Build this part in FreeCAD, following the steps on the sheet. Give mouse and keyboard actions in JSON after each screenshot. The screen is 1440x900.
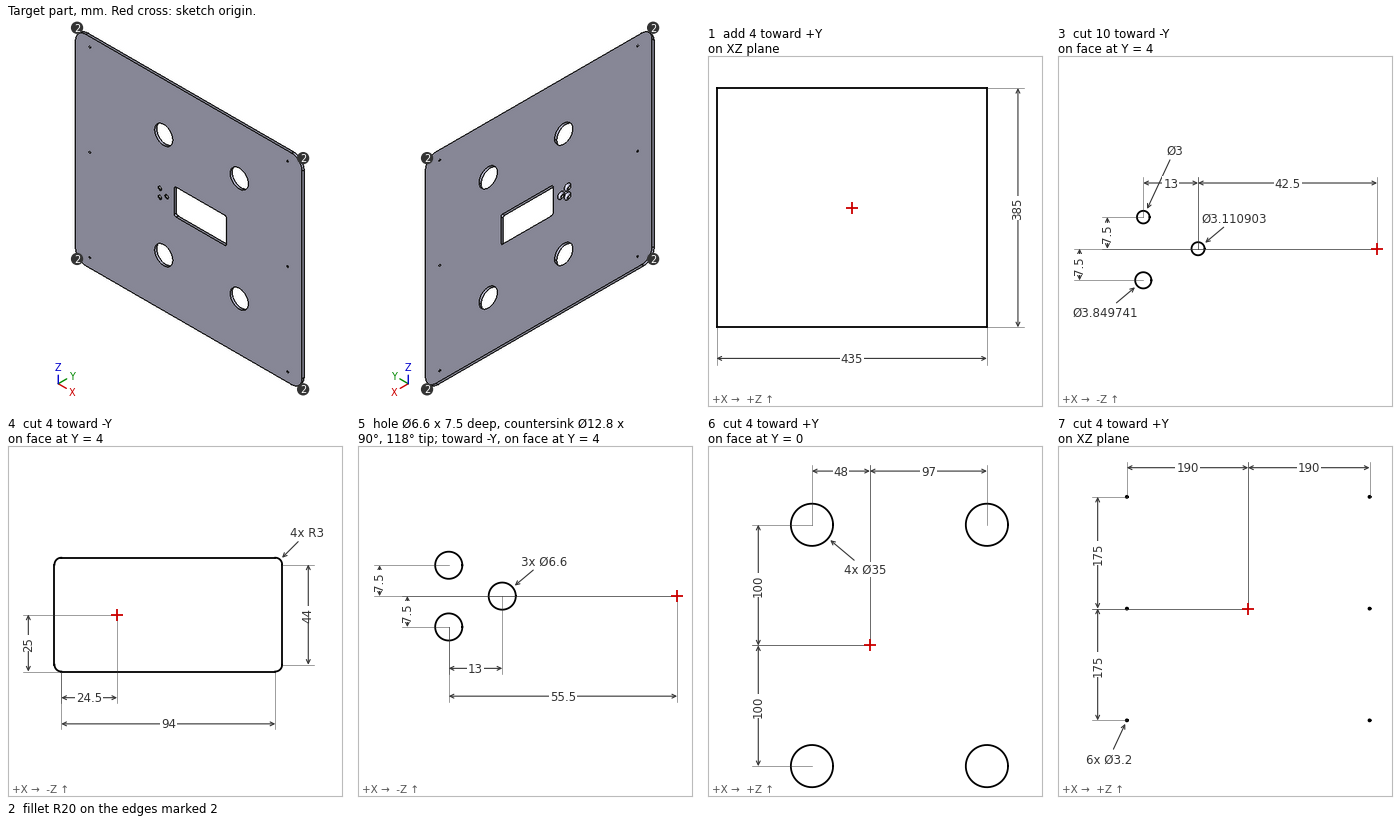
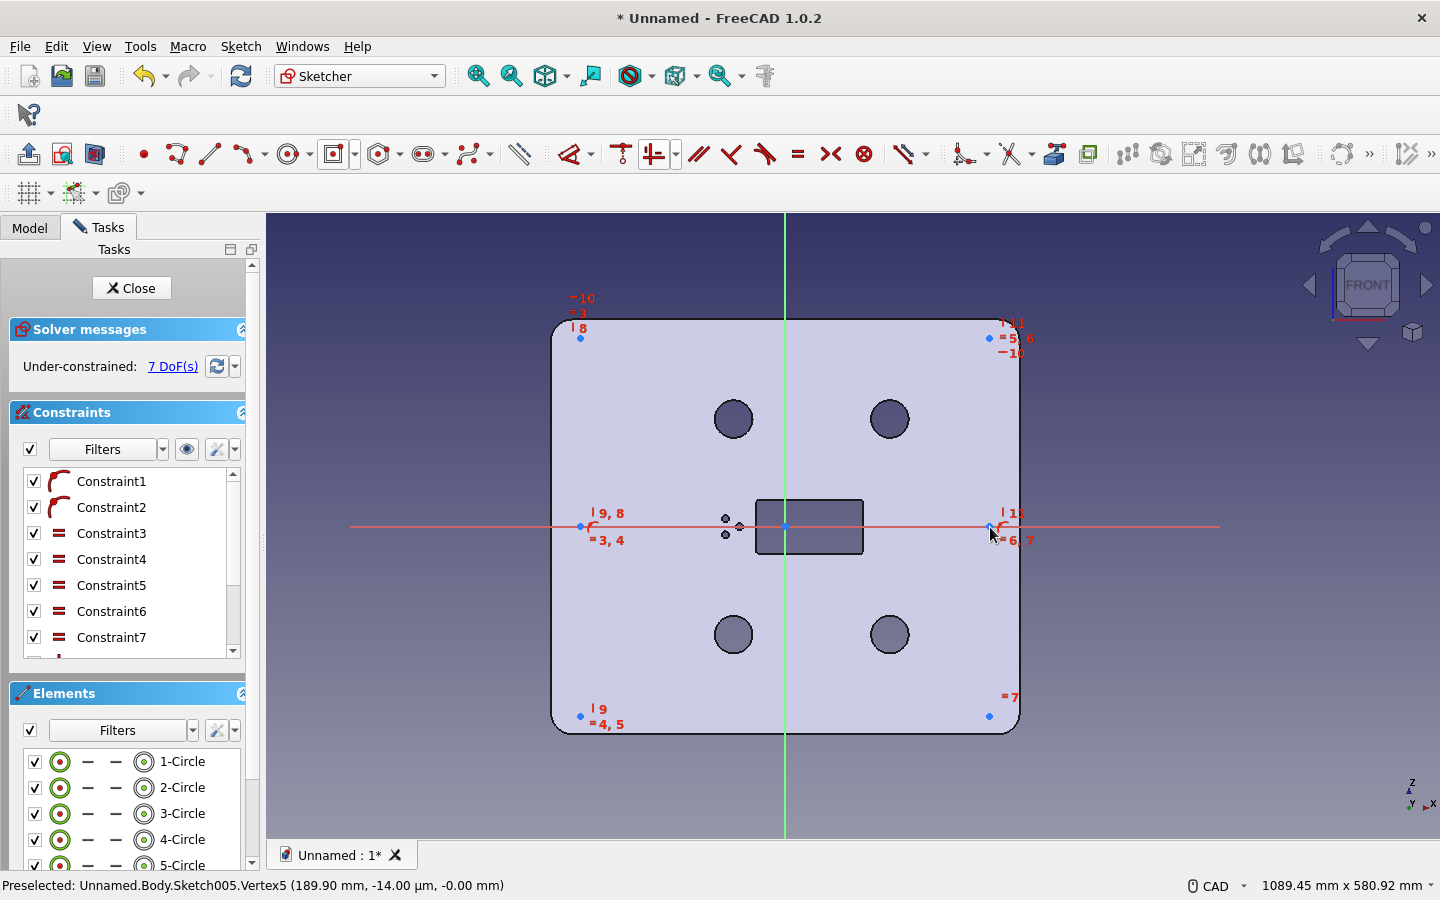
{"action": "left_click", "coordinate": [990, 527]}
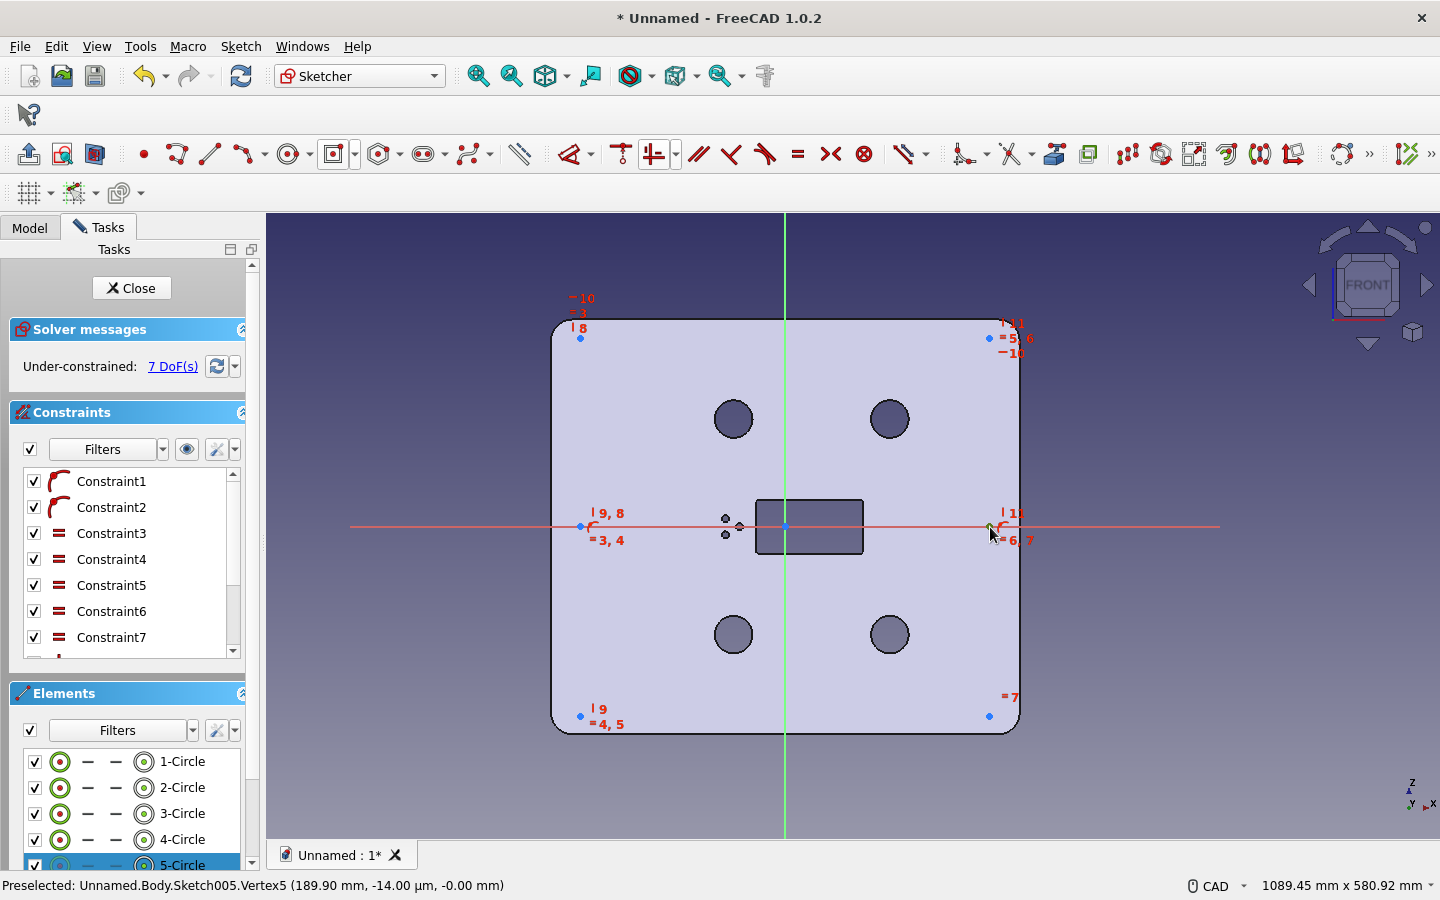
{"action": "left_click", "coordinate": [990, 717]}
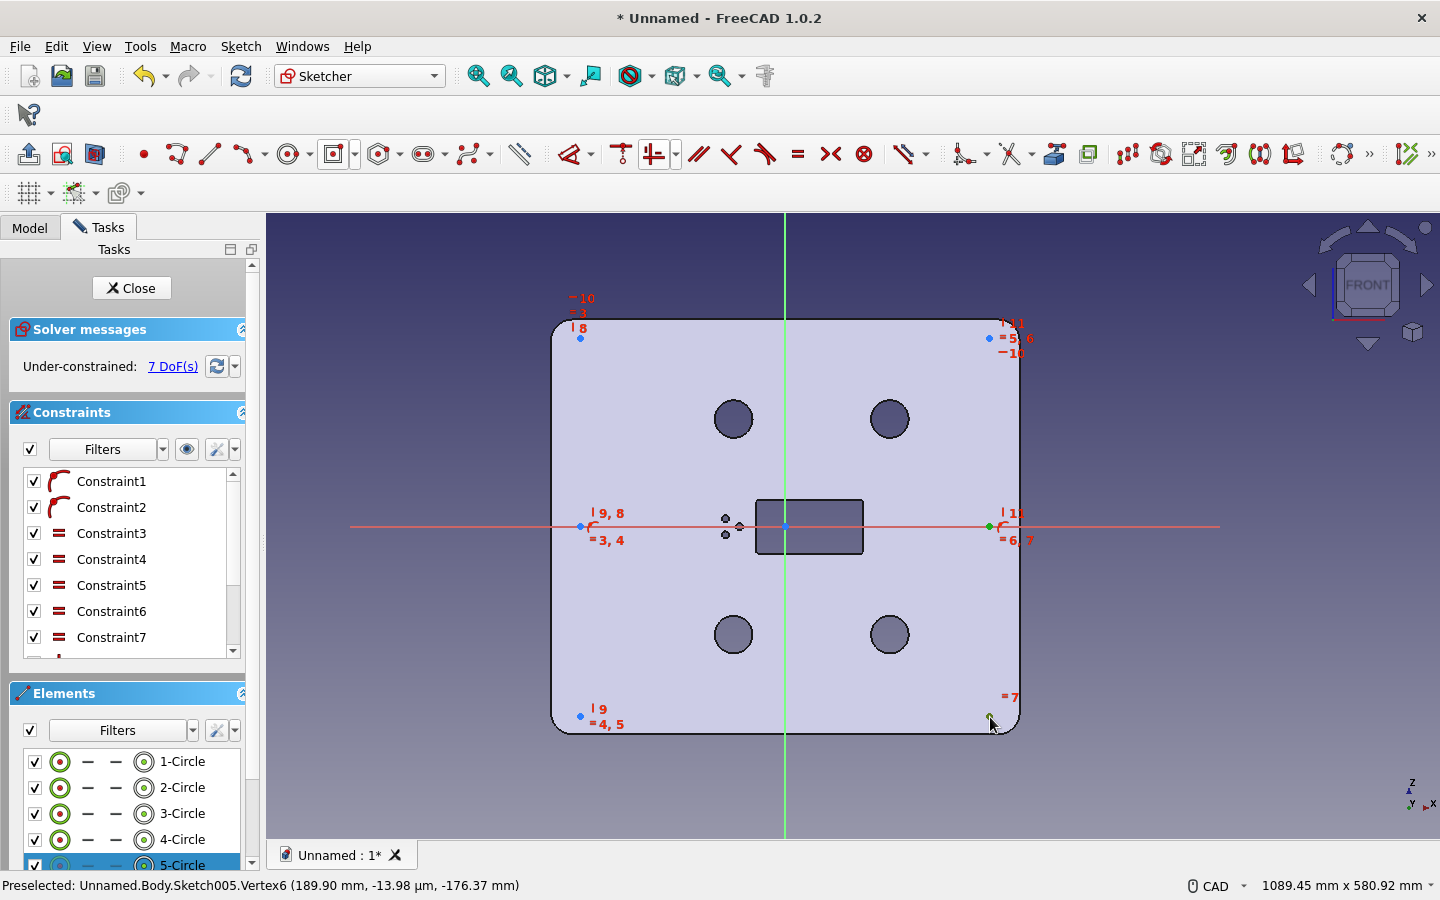
{"action": "key", "text": "v"}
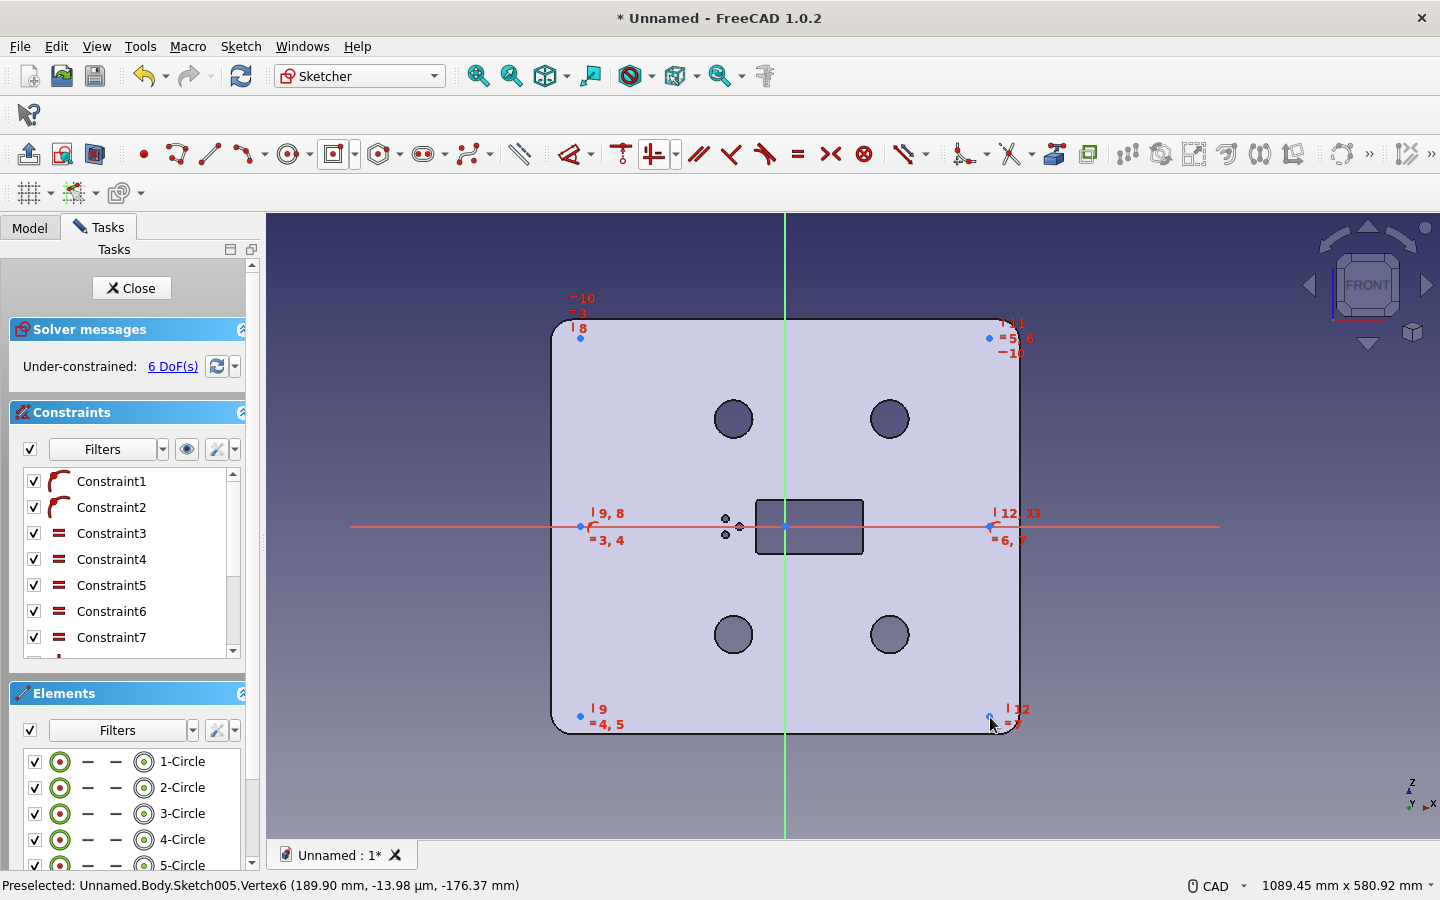
{"action": "left_click", "coordinate": [581, 717]}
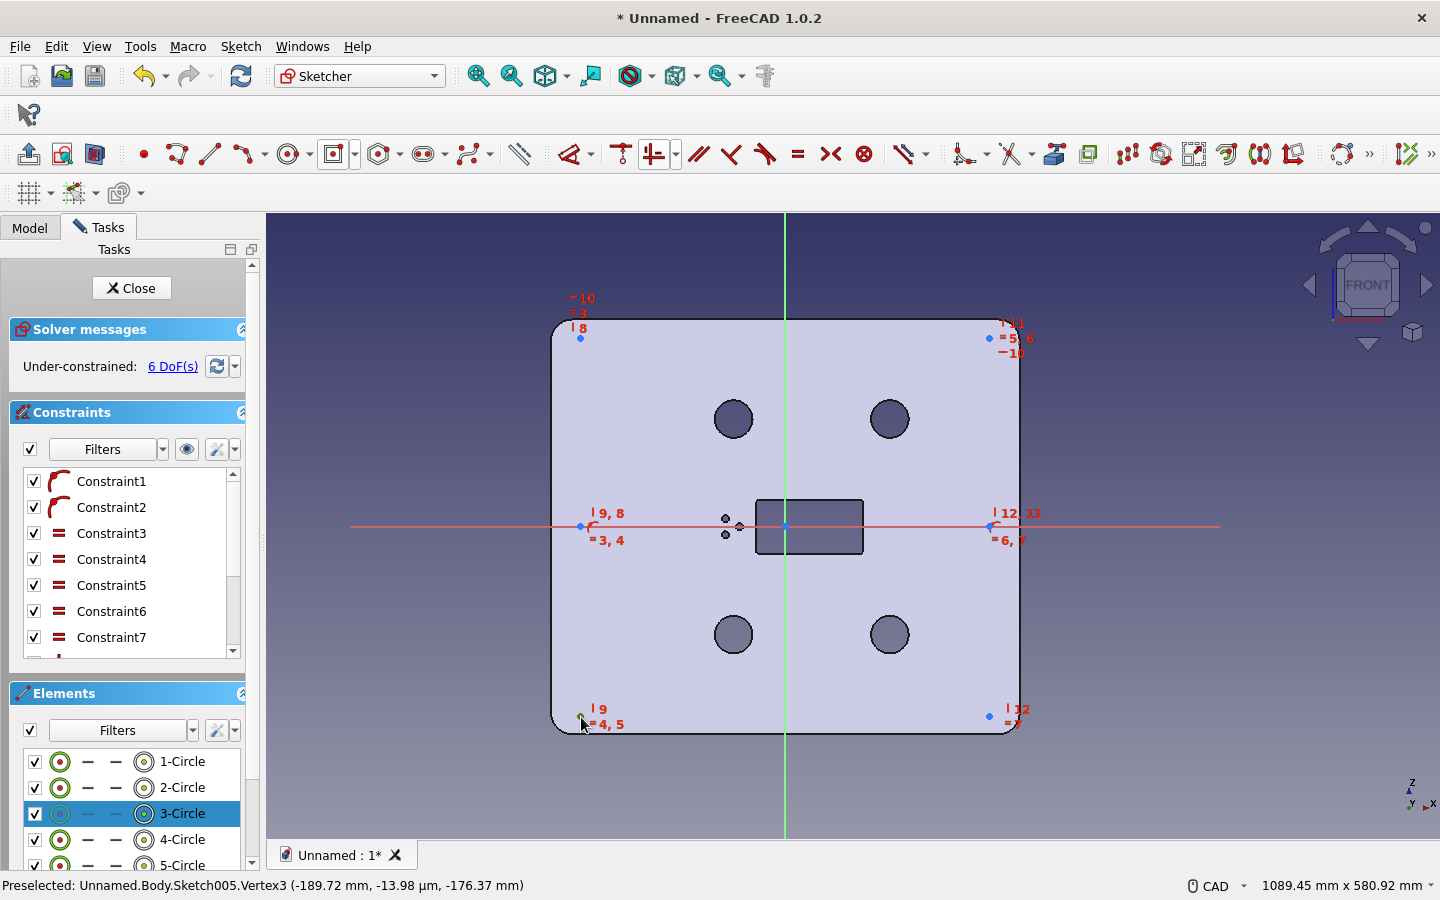
{"action": "left_click", "coordinate": [990, 717]}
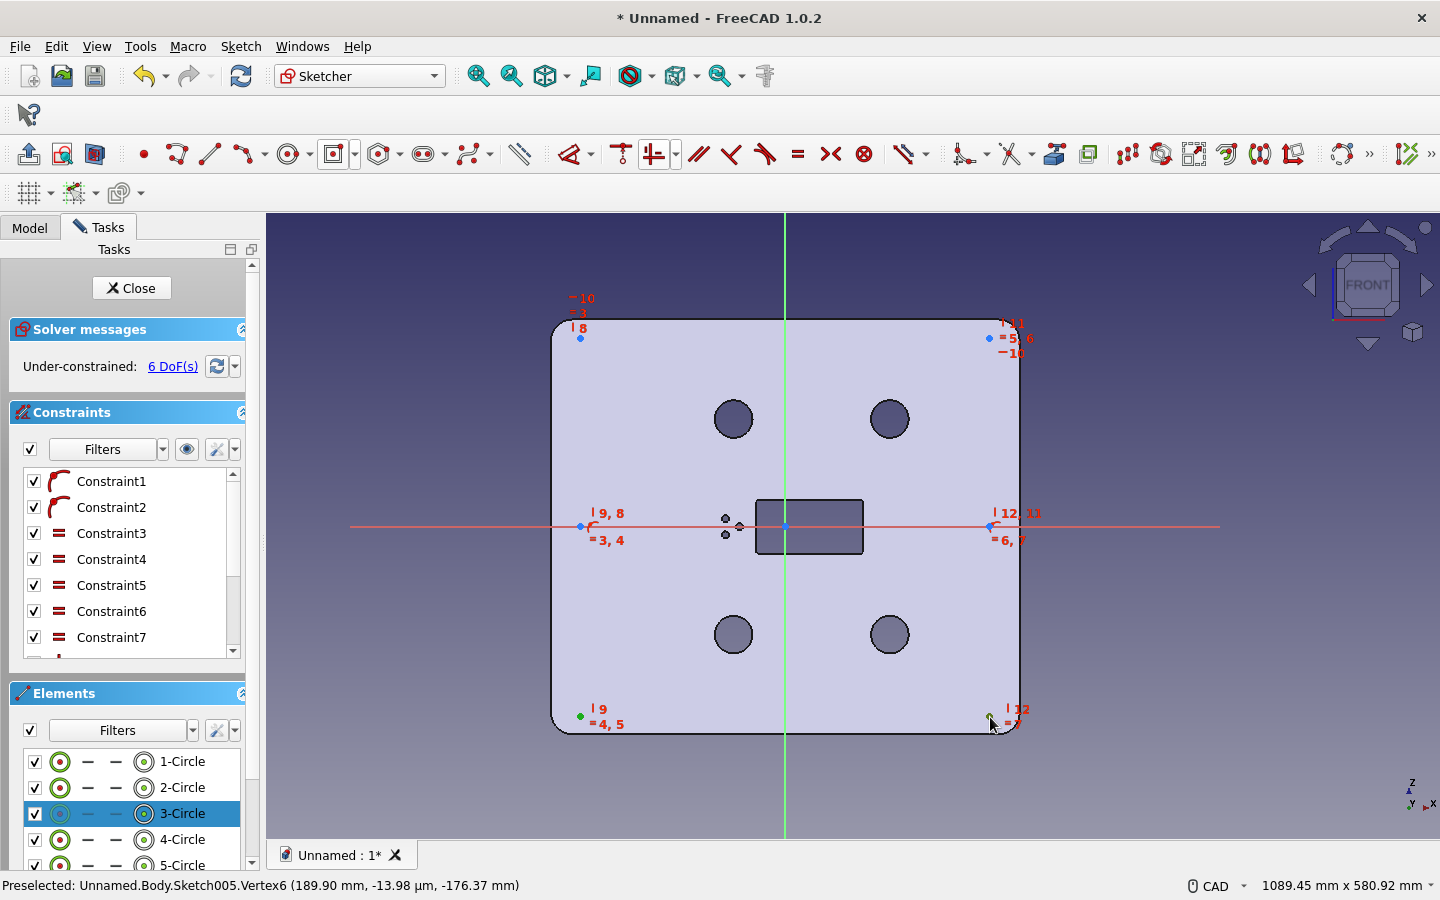
{"action": "left_click", "coordinate": [676, 154]}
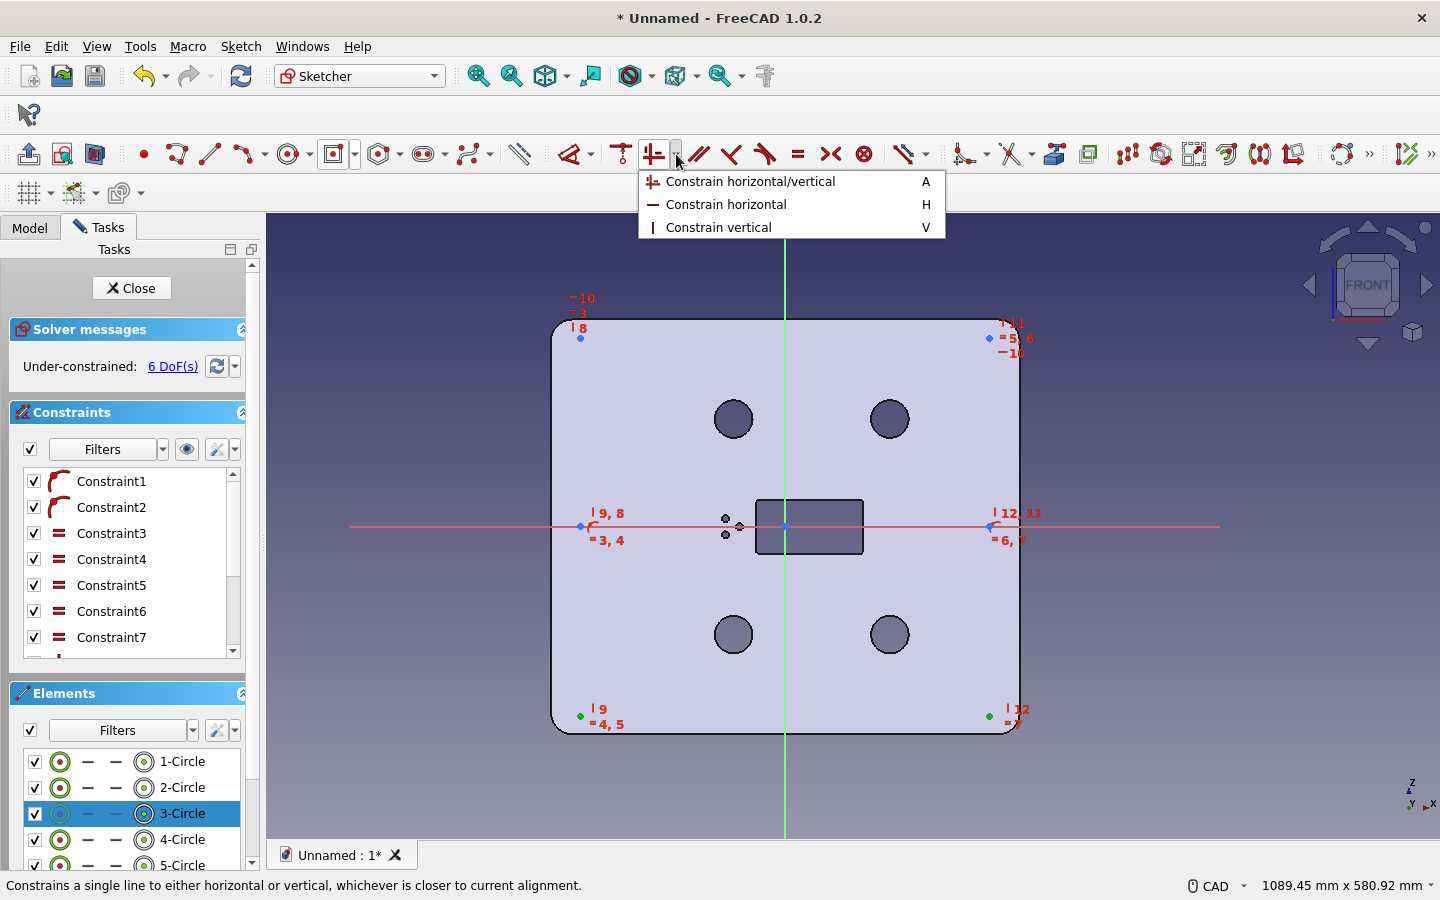
{"action": "left_click", "coordinate": [792, 204]}